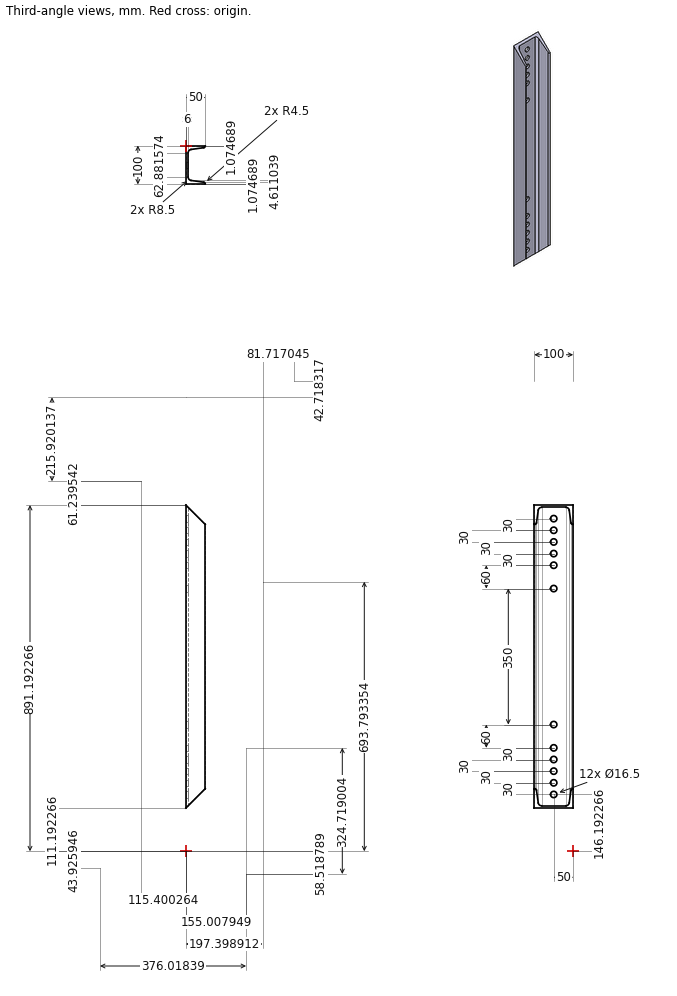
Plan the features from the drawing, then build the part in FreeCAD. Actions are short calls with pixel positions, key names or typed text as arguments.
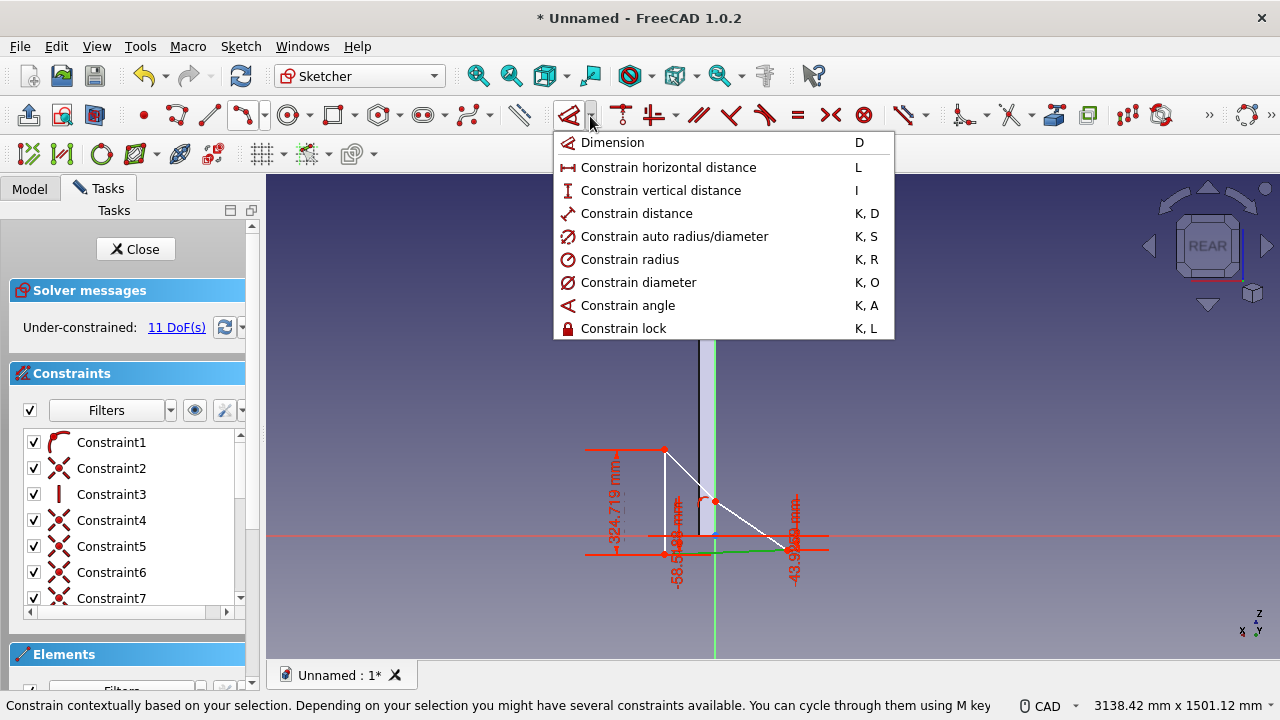
click(724, 168)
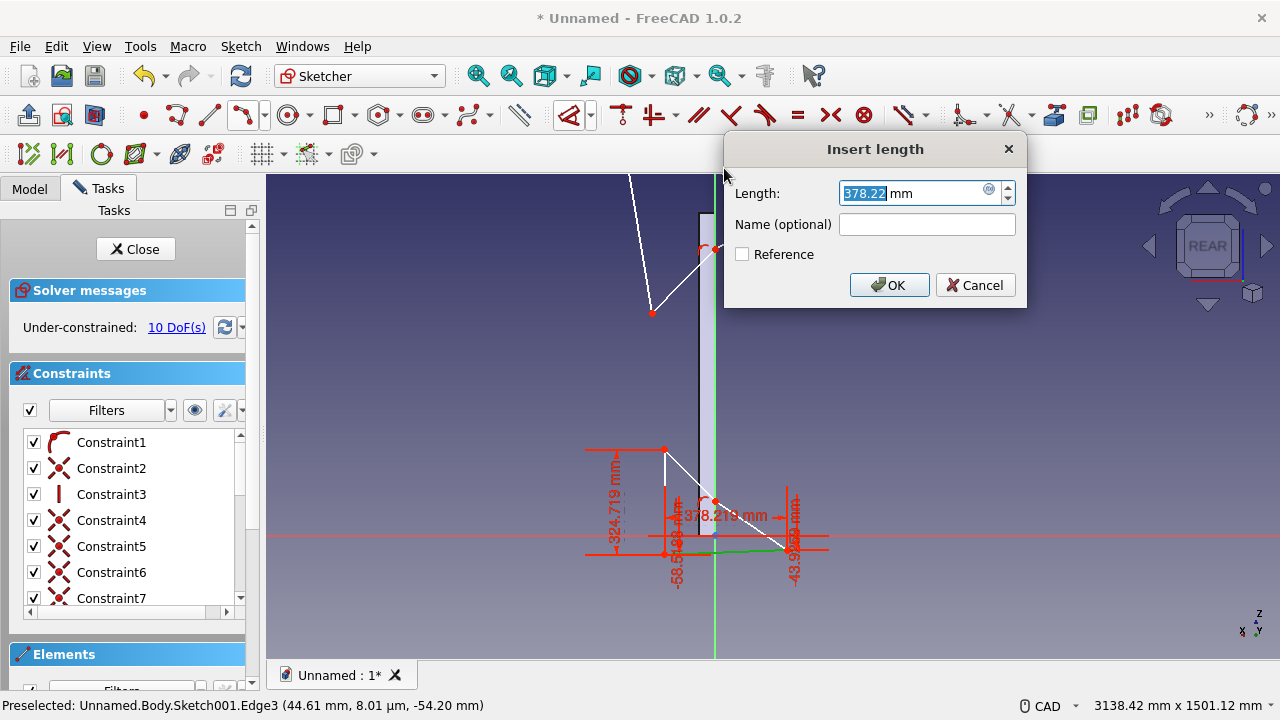
text(376.01839)
key(Return)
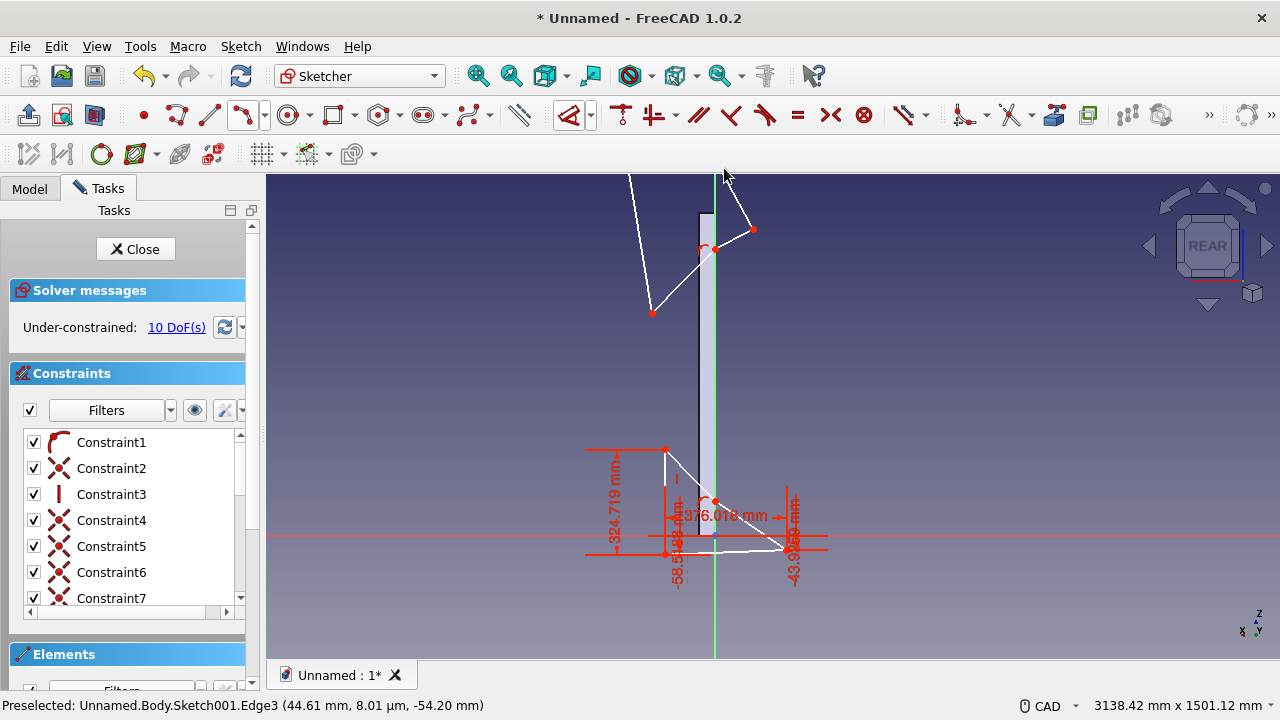
scroll(727, 243, up, 4)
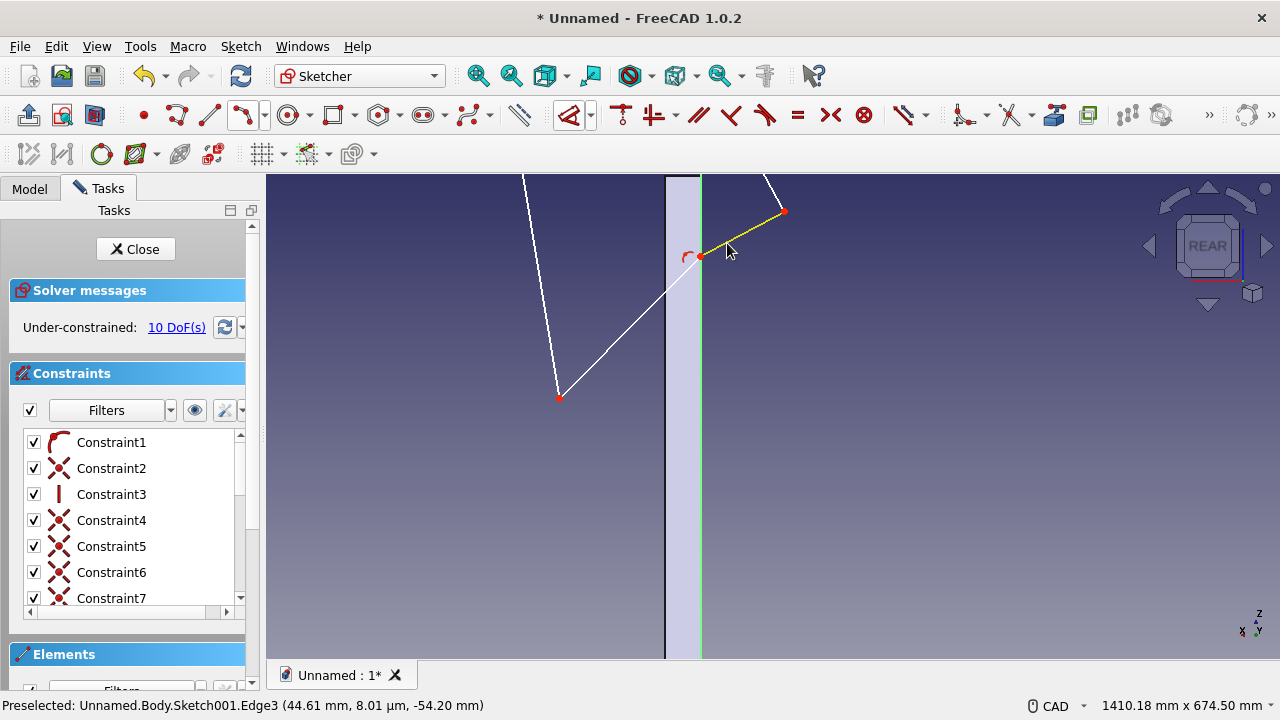
click(726, 243)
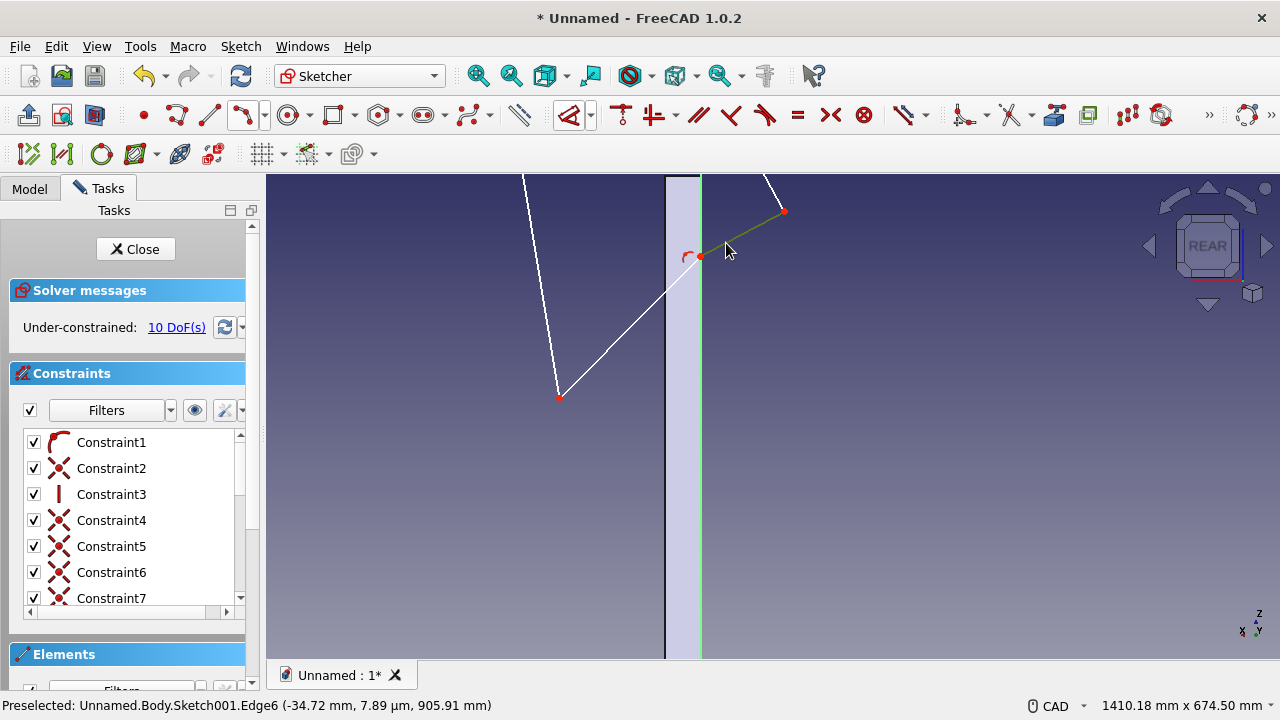
key(i)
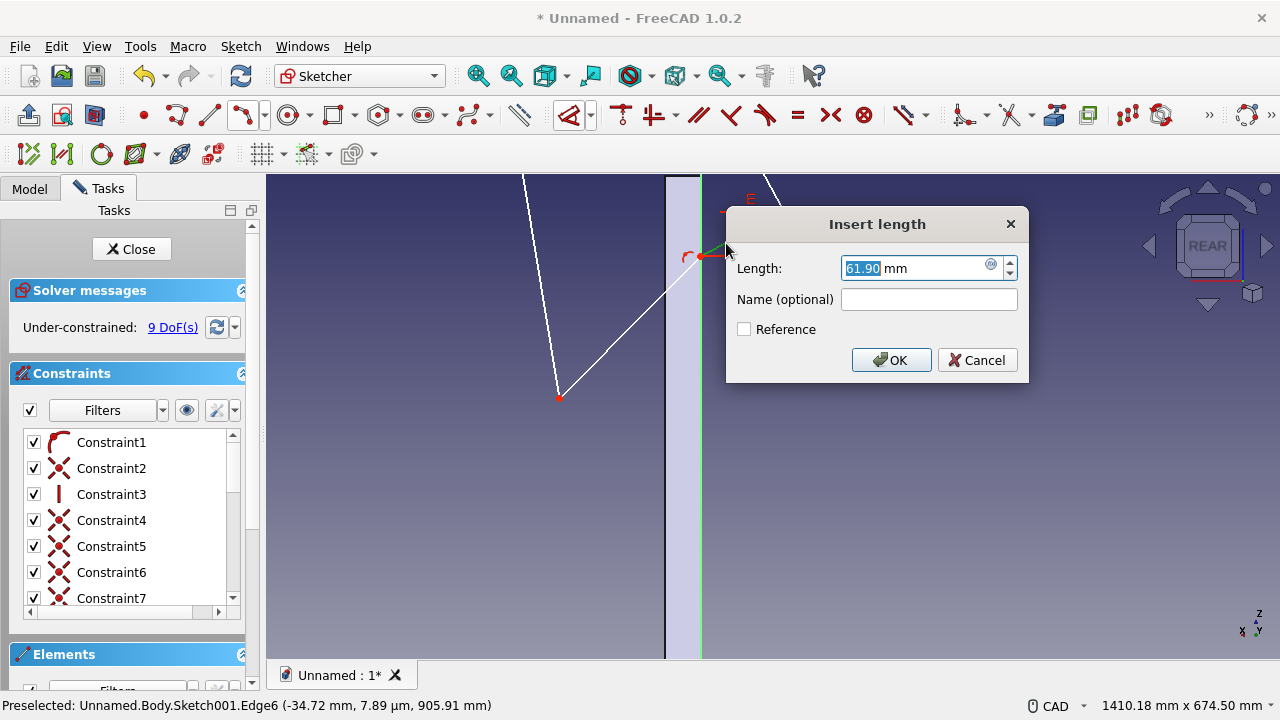
text(61.239542)
key(Return)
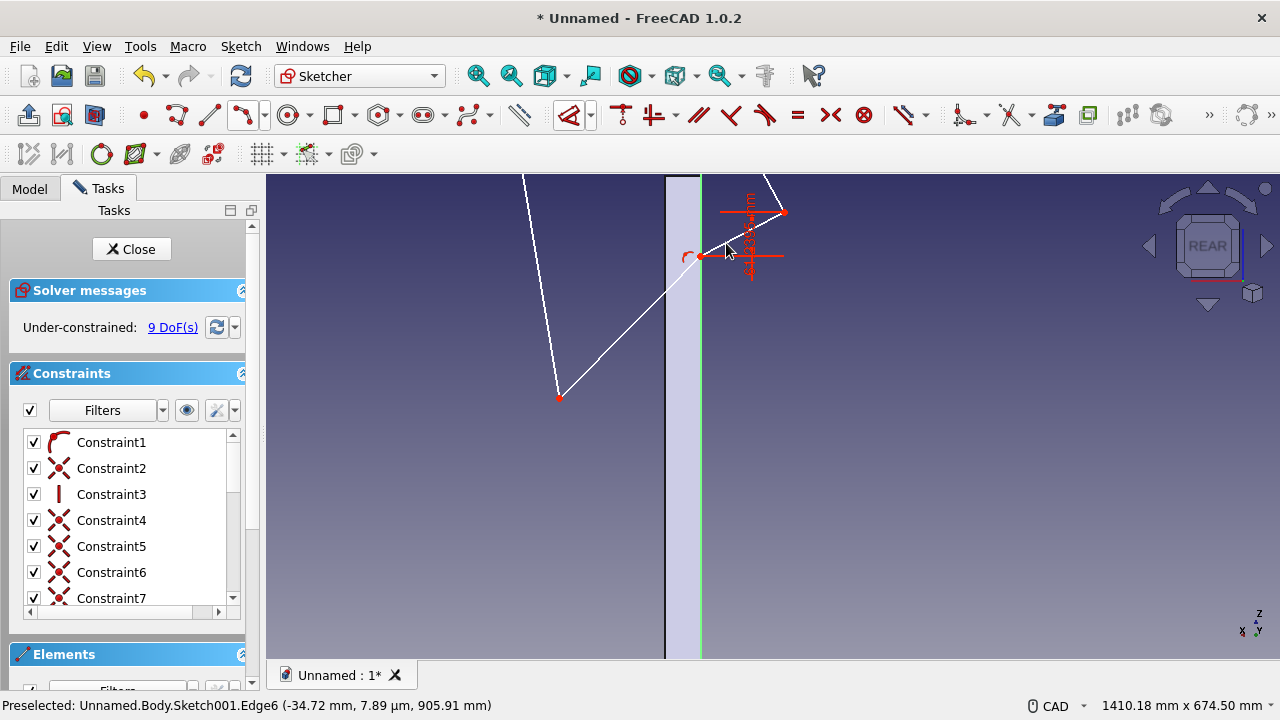
scroll(715, 389, down, 6)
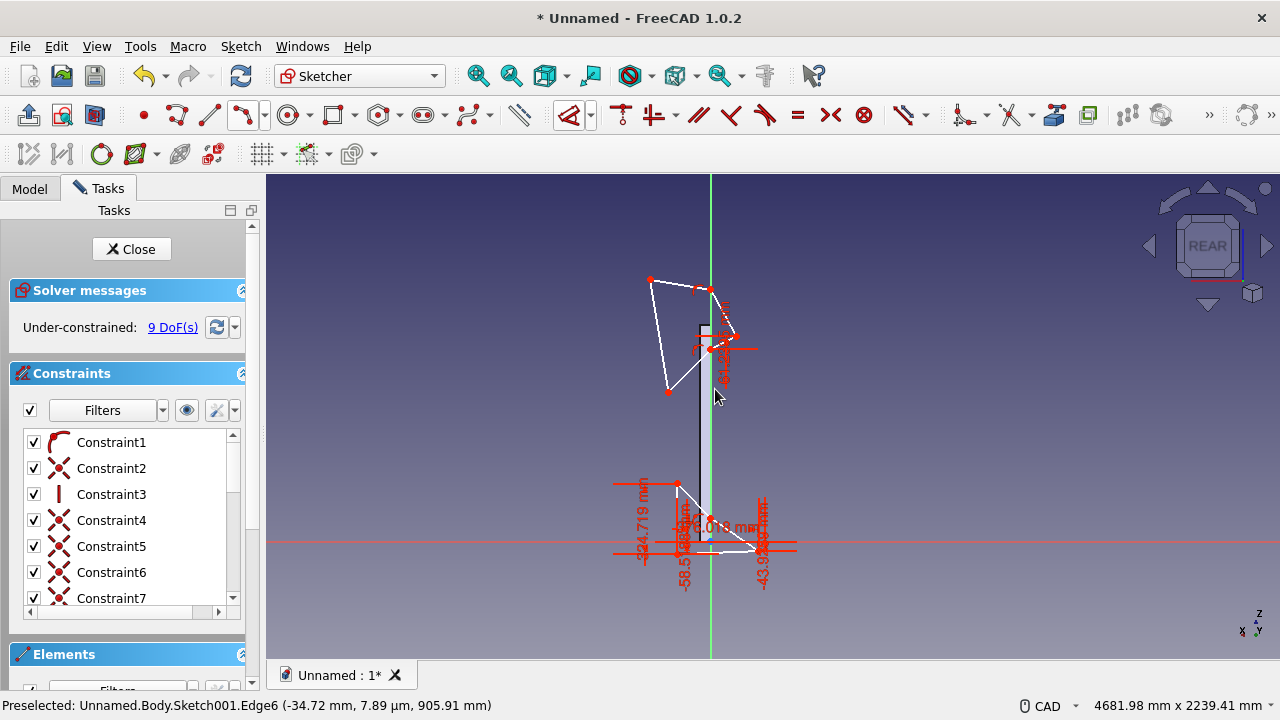
scroll(693, 287, up, 8)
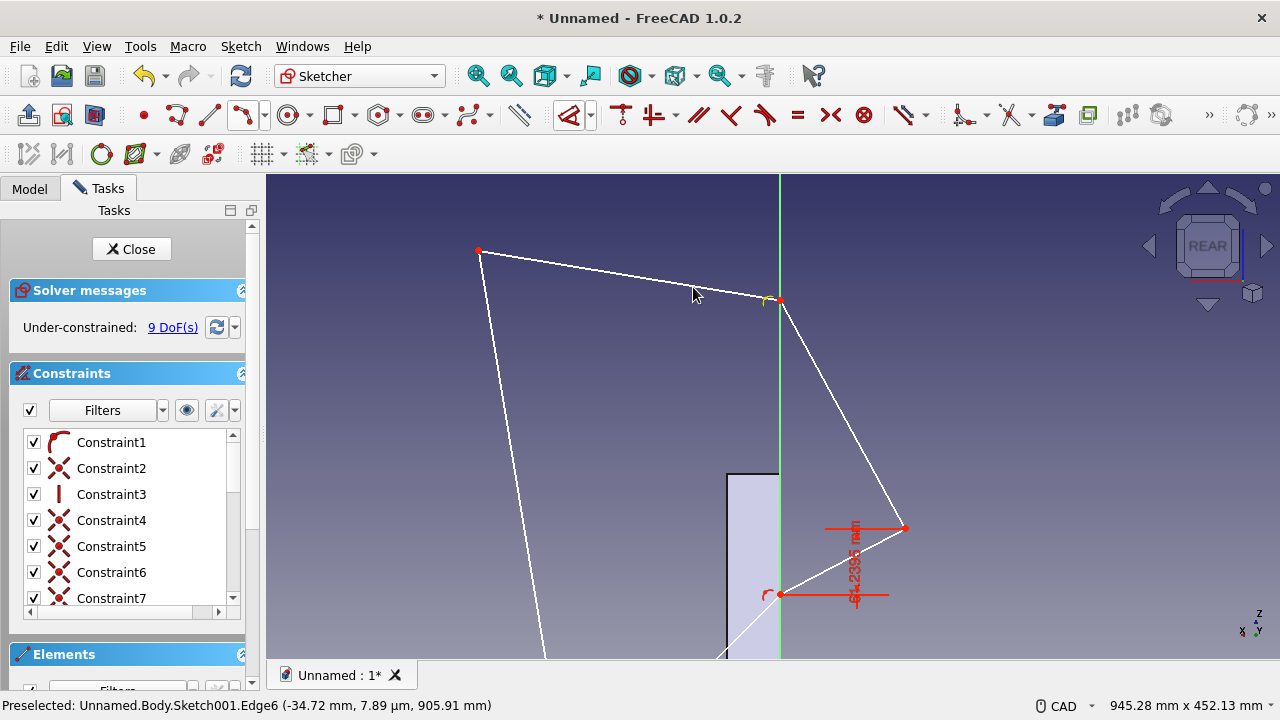
click(690, 286)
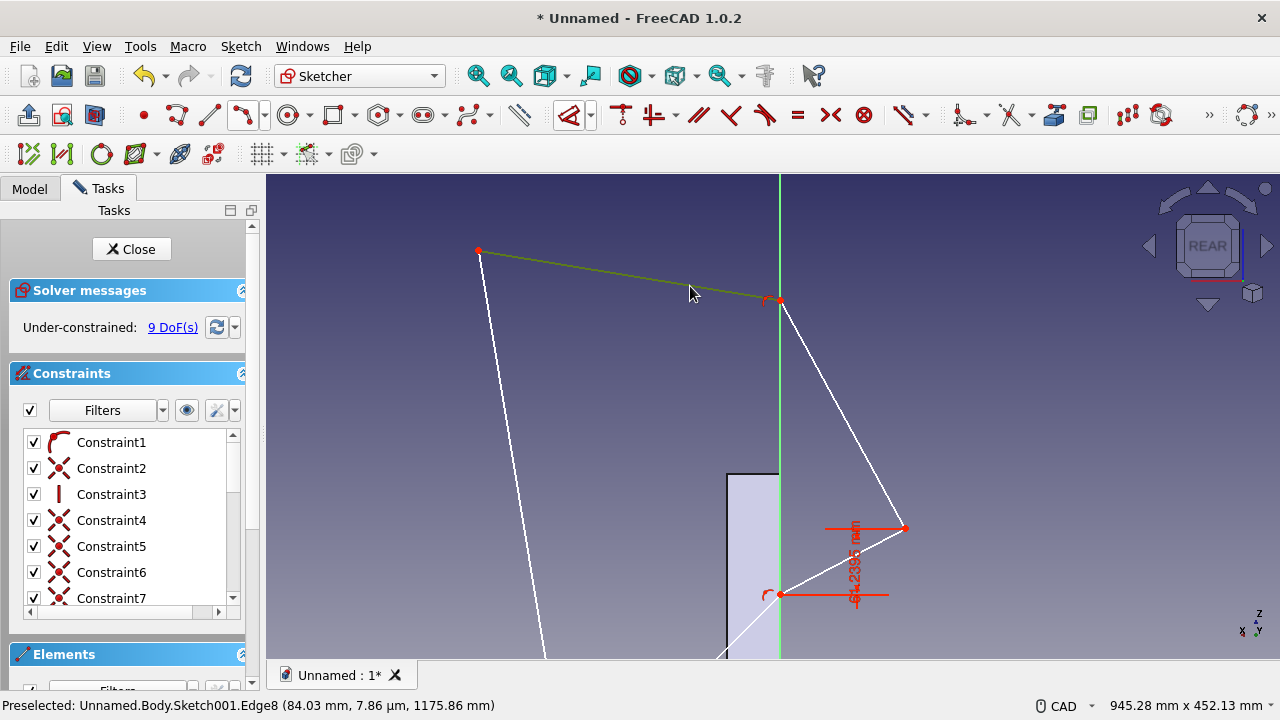
key(i)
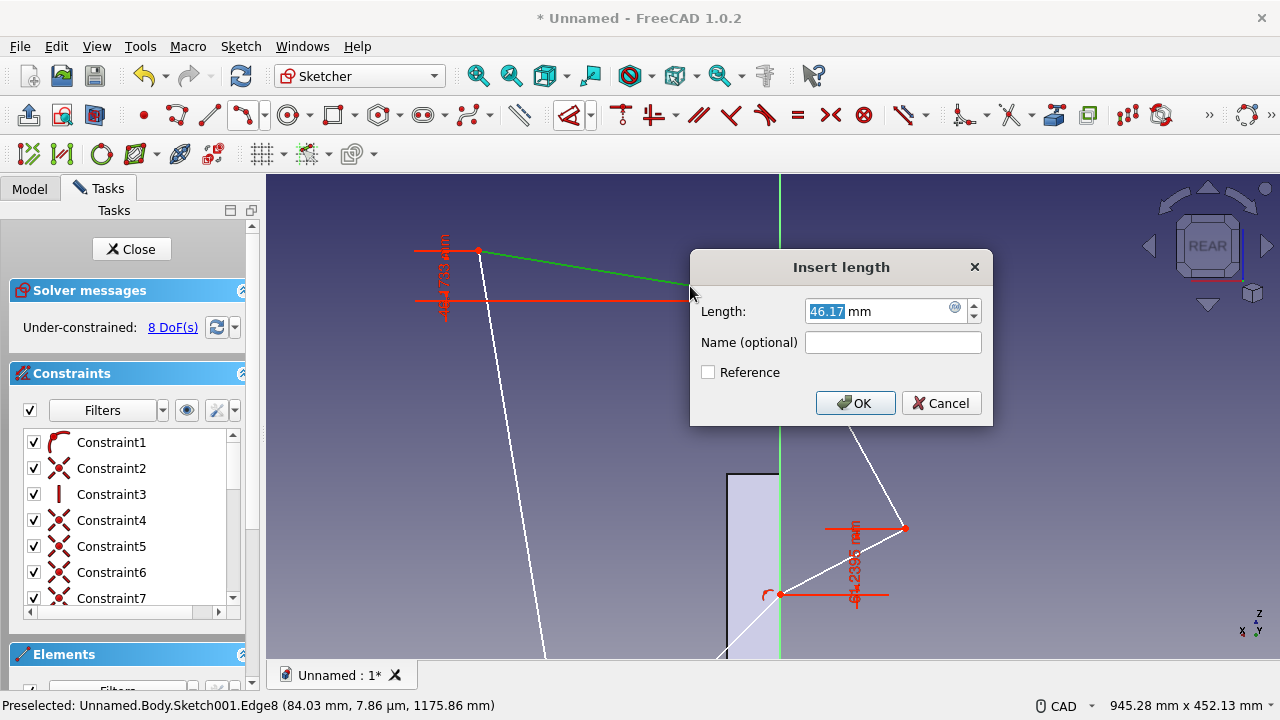
text(42.718317)
key(Return)